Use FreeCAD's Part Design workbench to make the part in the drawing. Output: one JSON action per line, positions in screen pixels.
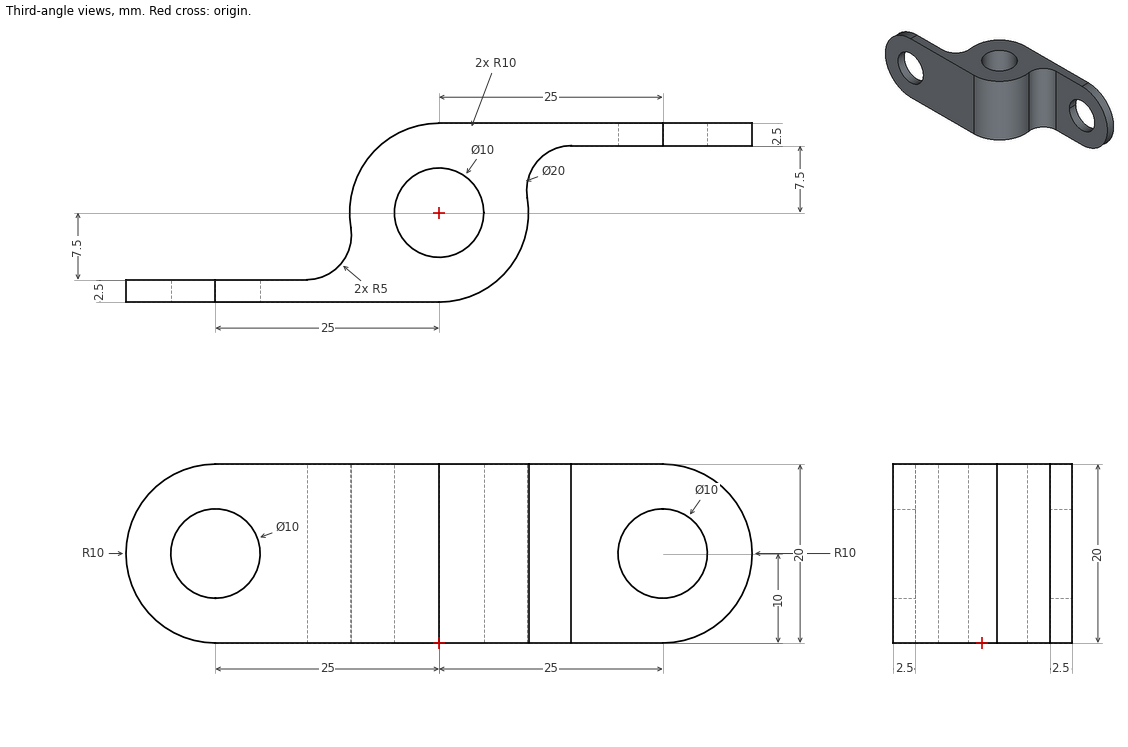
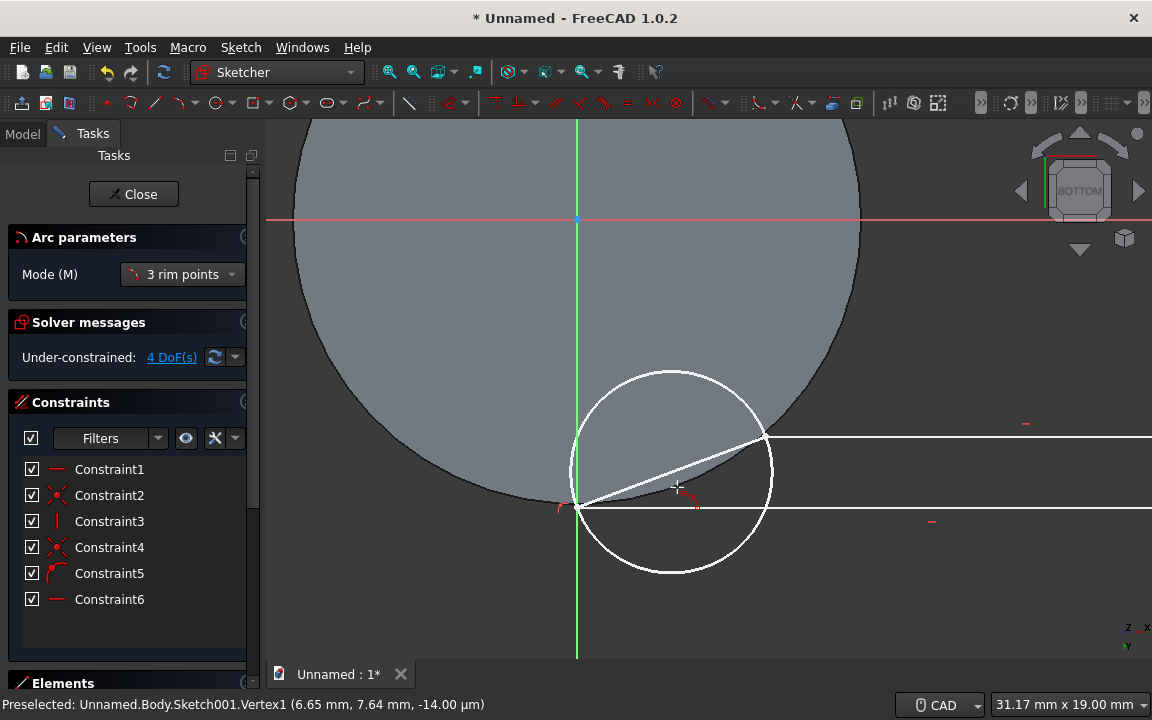
{"action": "left_click", "coordinate": [678, 486]}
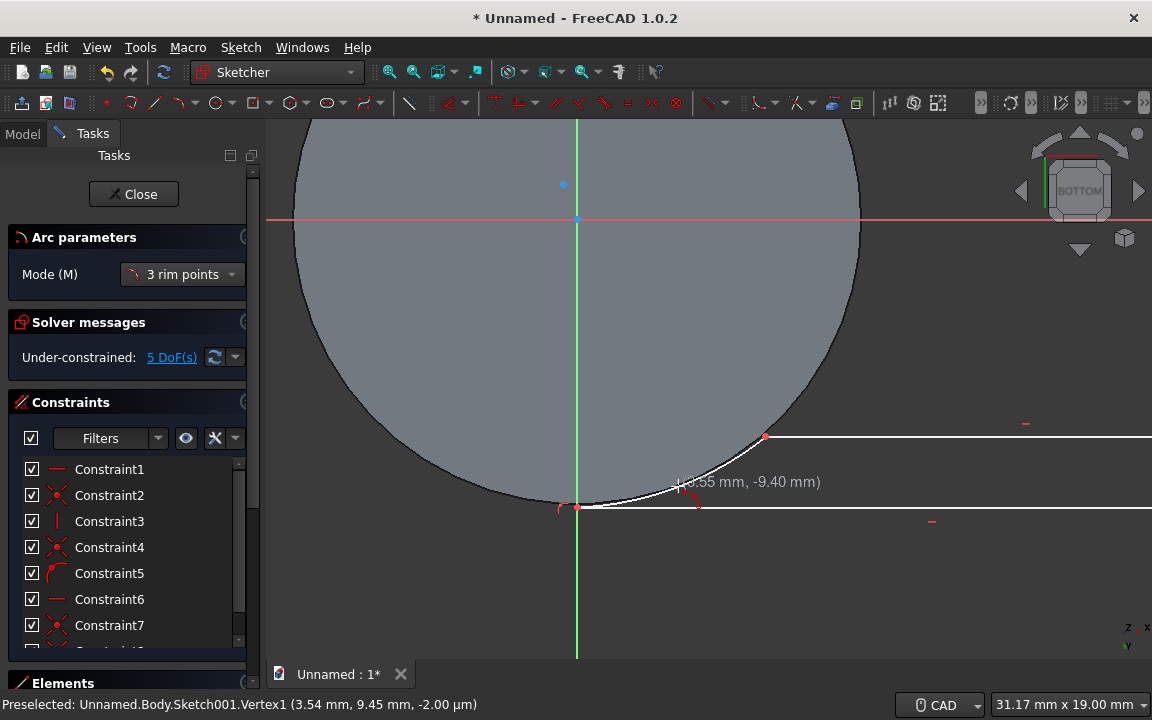
{"action": "key", "text": "g m"}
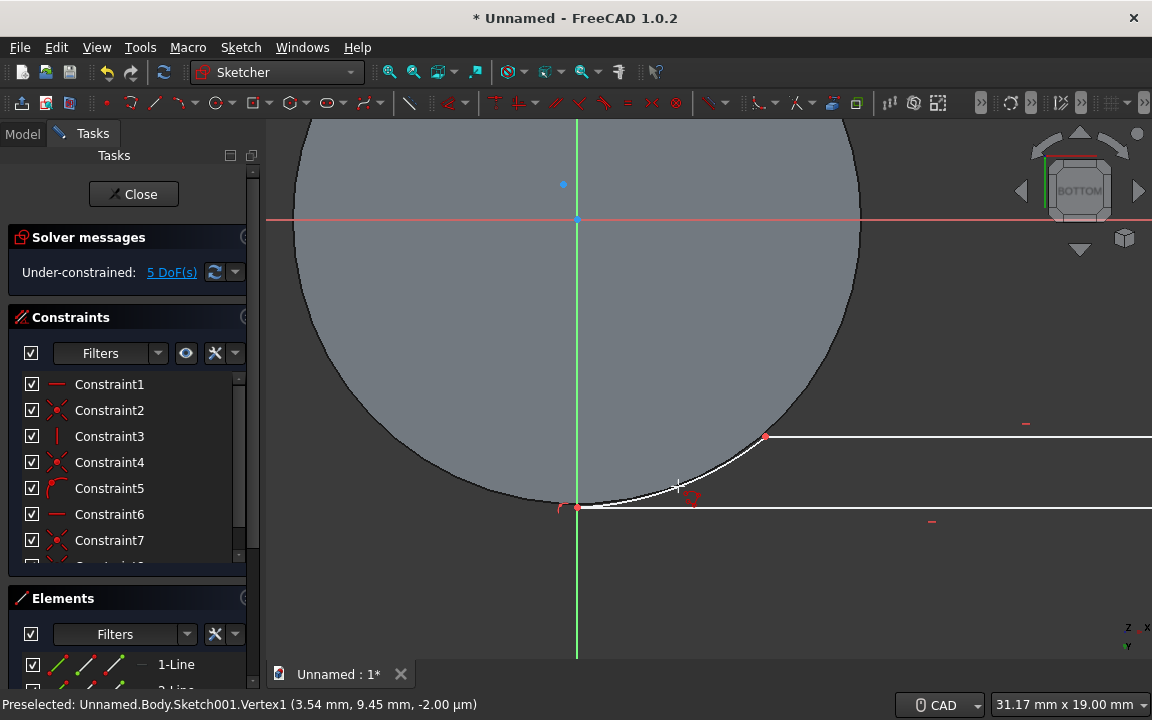
{"action": "scroll", "coordinate": [677, 487], "scroll_direction": "down", "scroll_amount": 5}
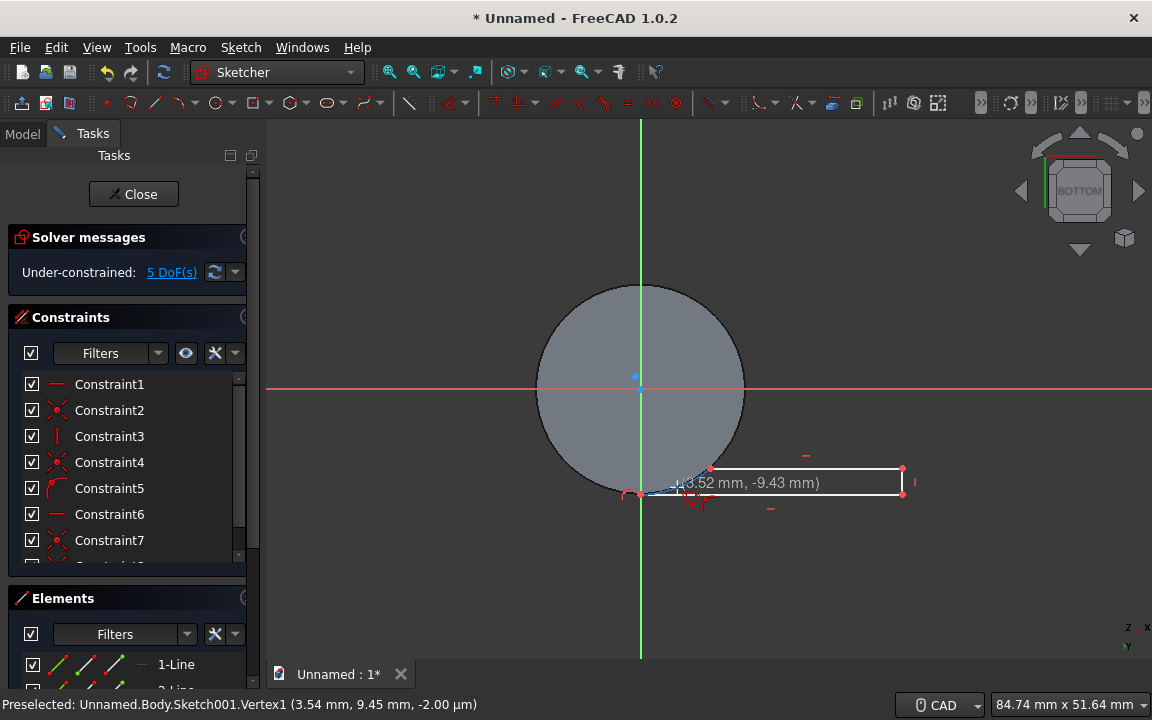
{"action": "left_click", "coordinate": [571, 311]}
{"action": "left_click", "coordinate": [379, 311]}
{"action": "left_click", "coordinate": [379, 285]}
{"action": "left_click", "coordinate": [641, 285]}
{"action": "right_click", "coordinate": [641, 285]}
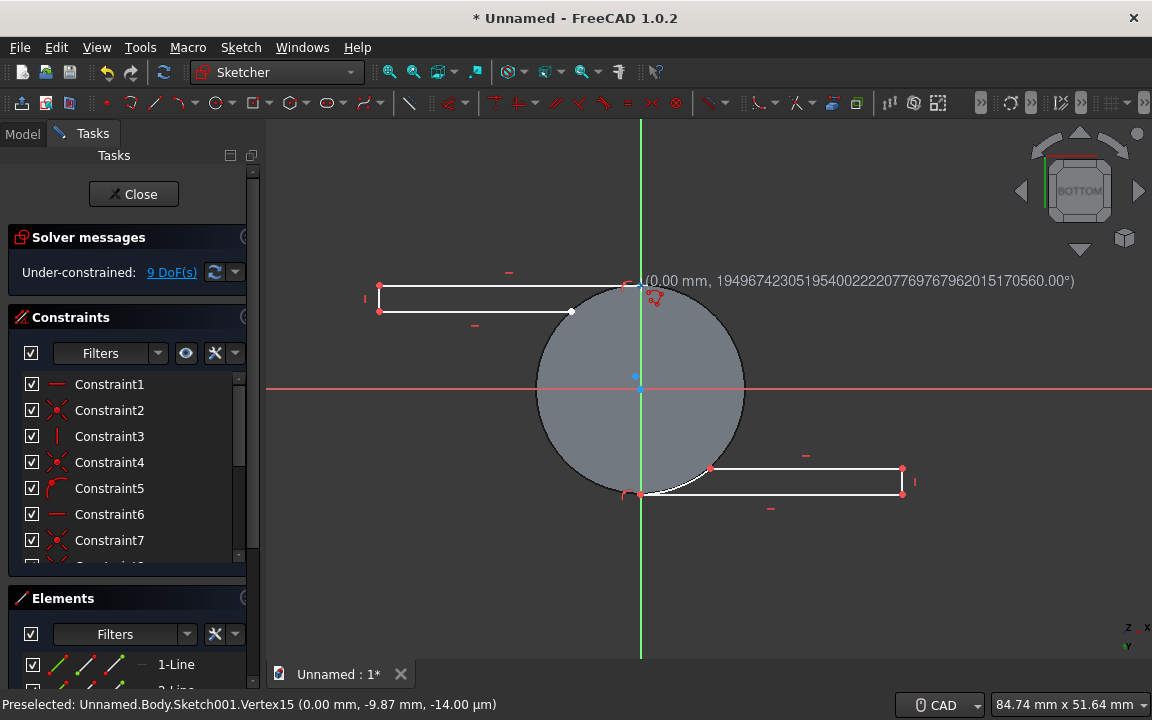
{"action": "key", "text": "g 3 a"}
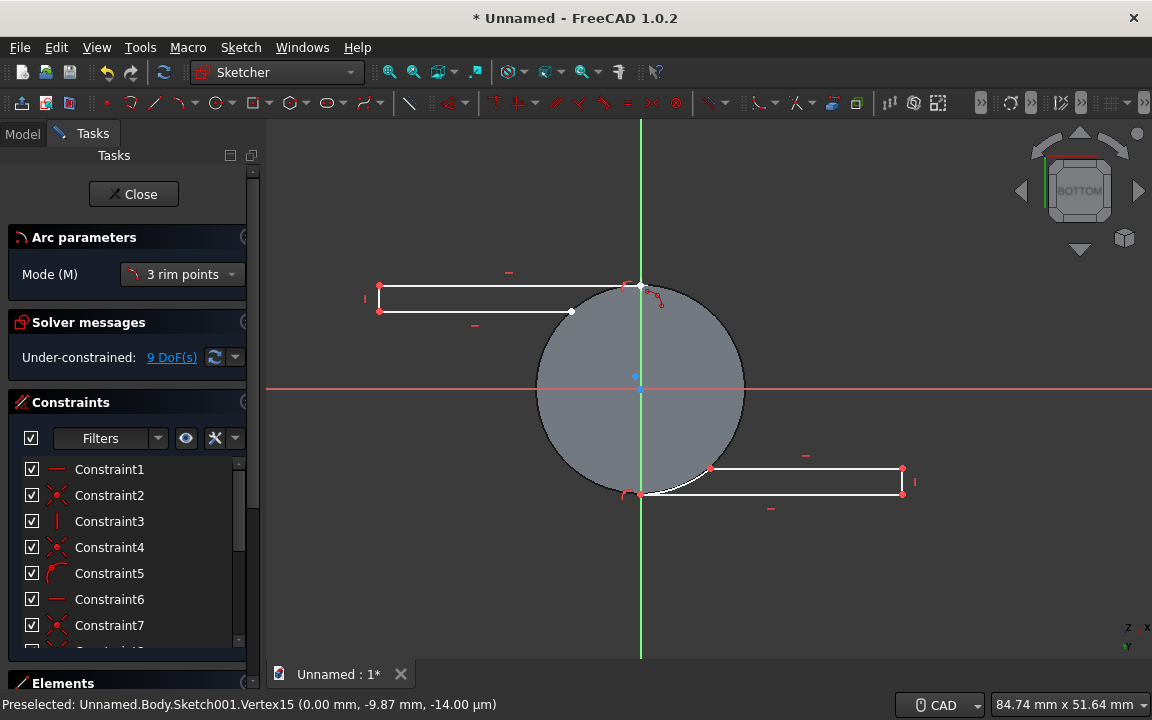
{"action": "left_click", "coordinate": [641, 286]}
{"action": "left_click", "coordinate": [571, 312]}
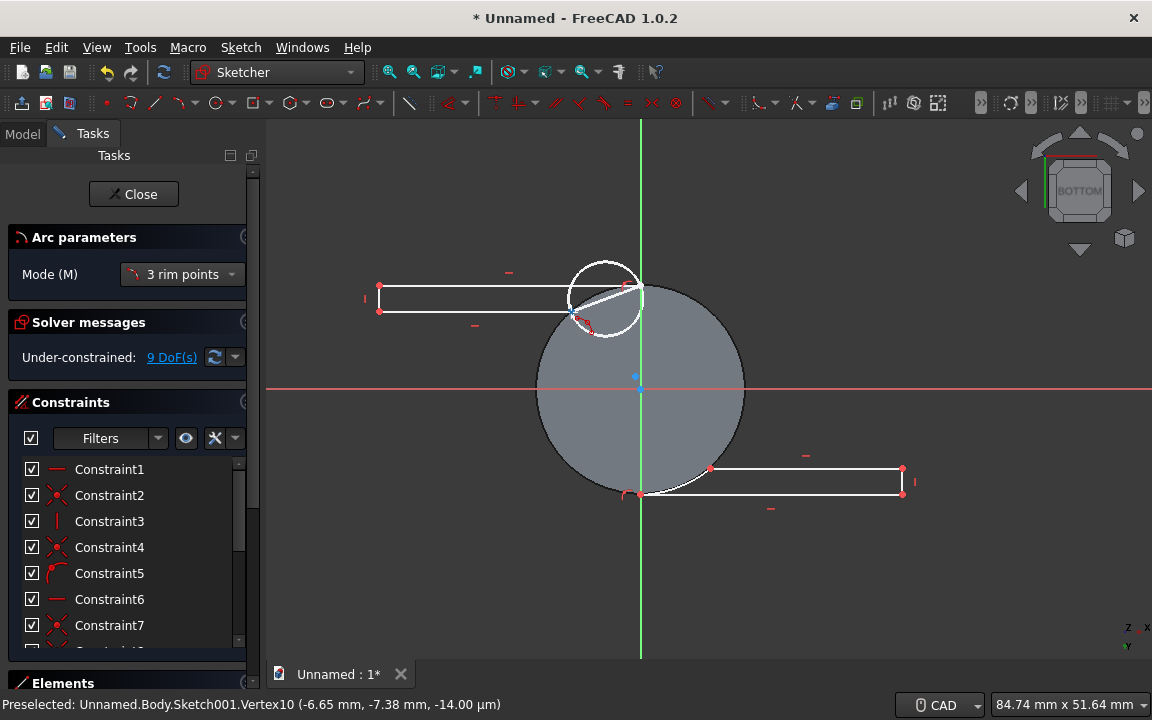
{"action": "scroll", "coordinate": [604, 291], "scroll_direction": "up", "scroll_amount": 5}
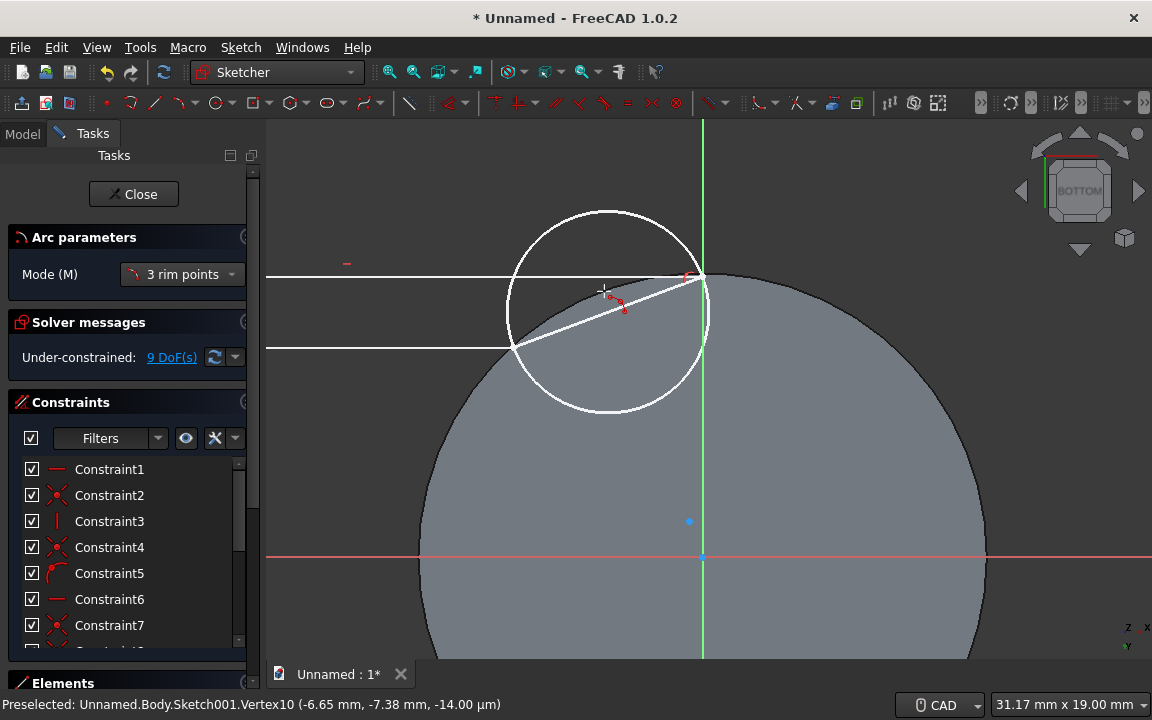
{"action": "left_click", "coordinate": [602, 291]}
{"action": "key", "text": "Escape"}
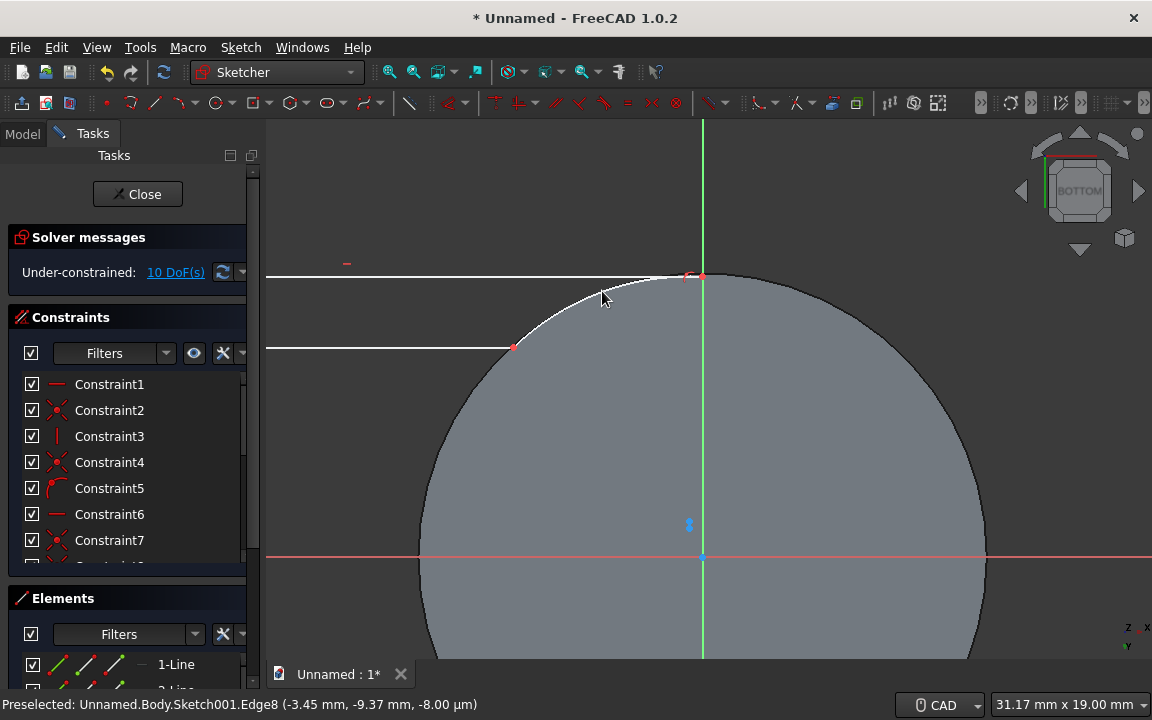
{"action": "scroll", "coordinate": [604, 291], "scroll_direction": "down", "scroll_amount": 5}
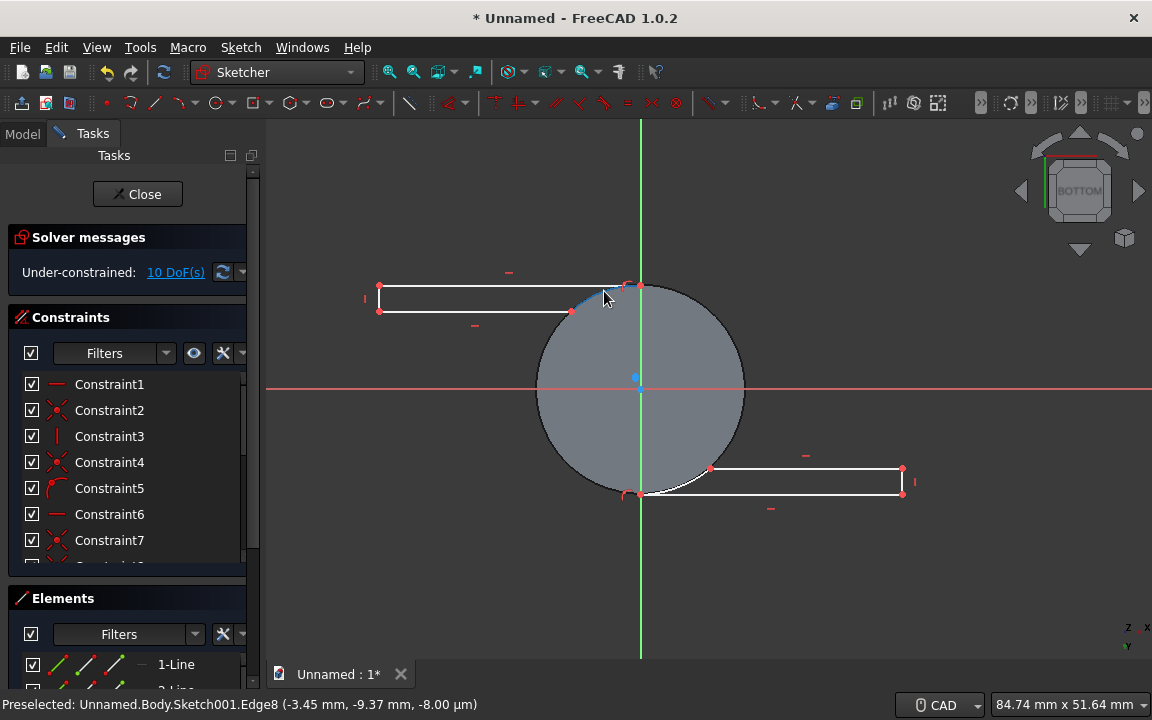
{"action": "left_click", "coordinate": [824, 495]}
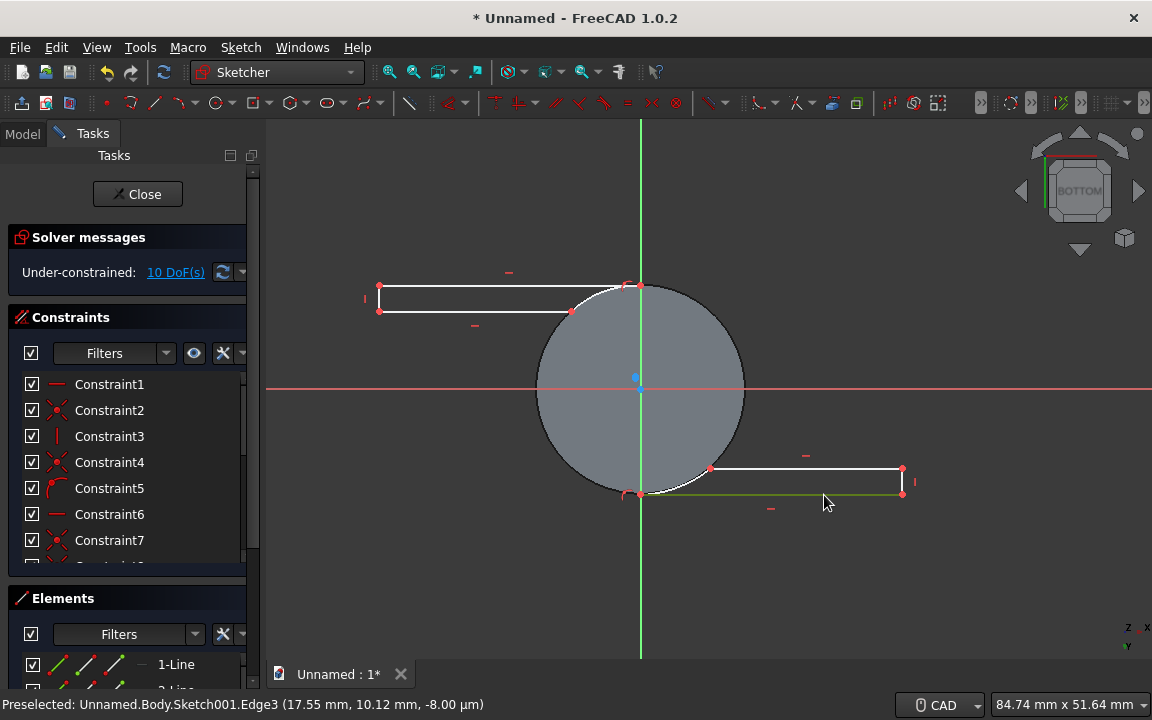
{"action": "left_click", "coordinate": [691, 481]}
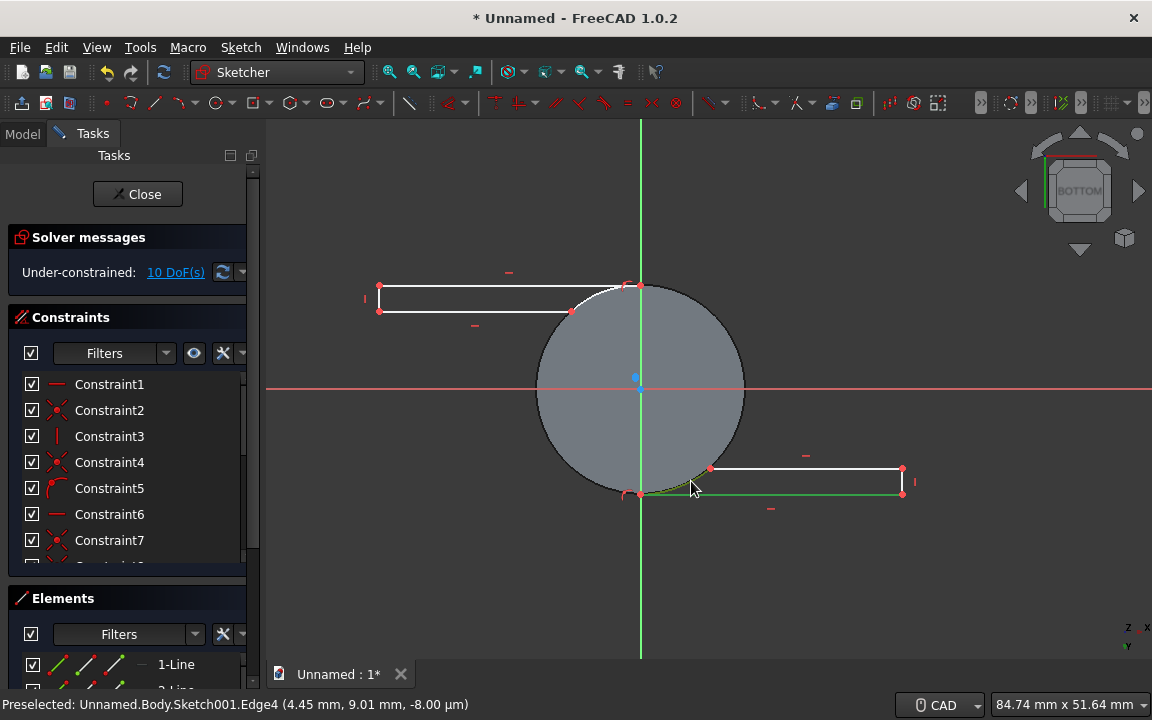
{"action": "left_click", "coordinate": [604, 104]}